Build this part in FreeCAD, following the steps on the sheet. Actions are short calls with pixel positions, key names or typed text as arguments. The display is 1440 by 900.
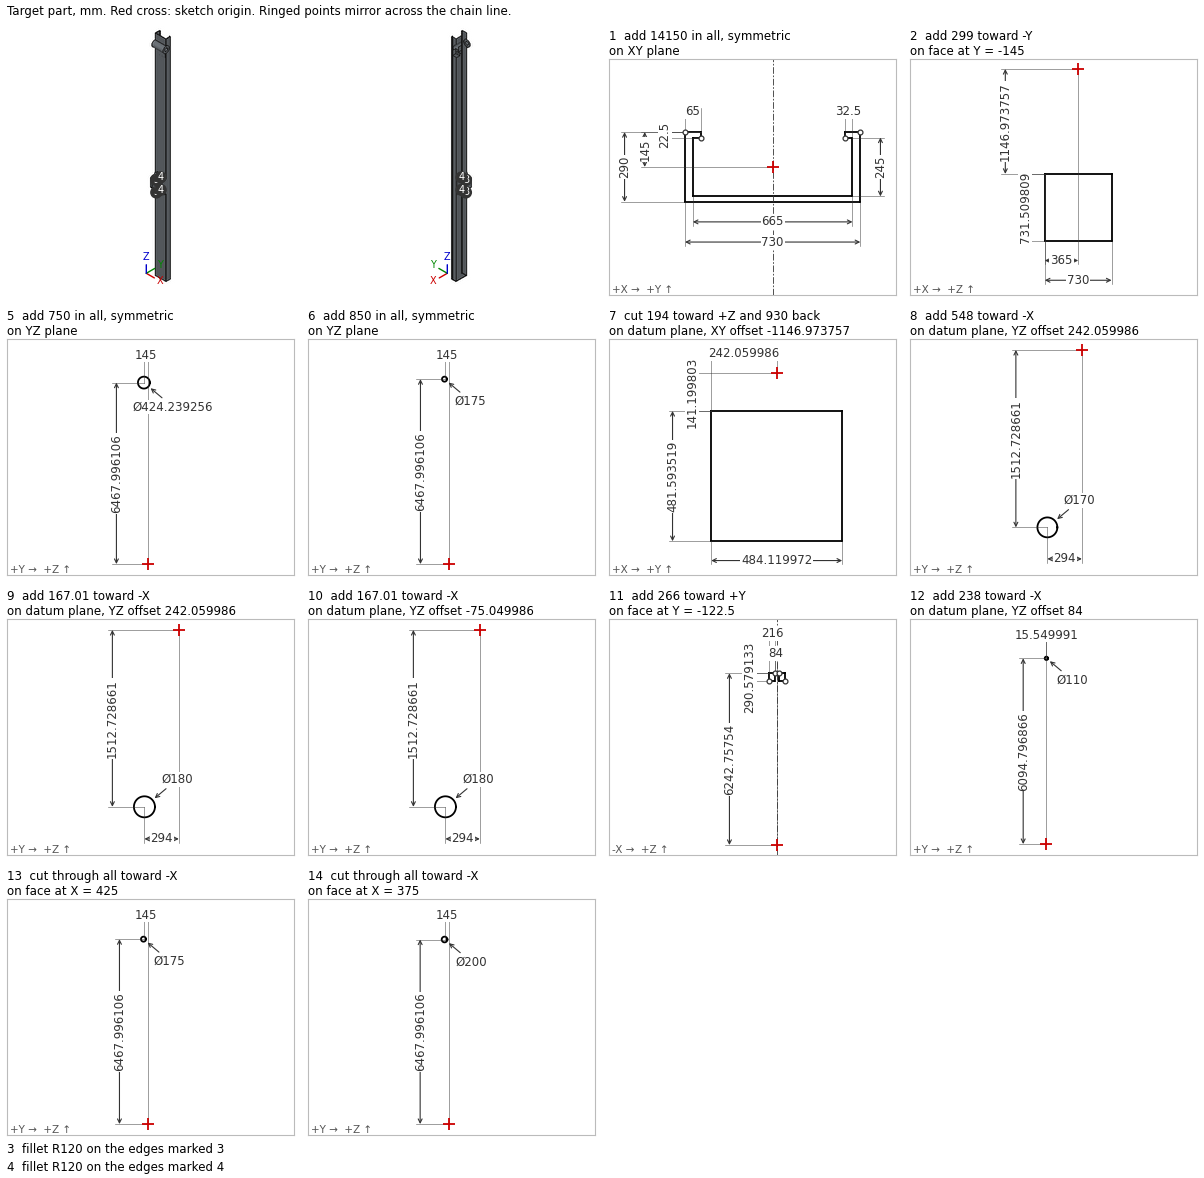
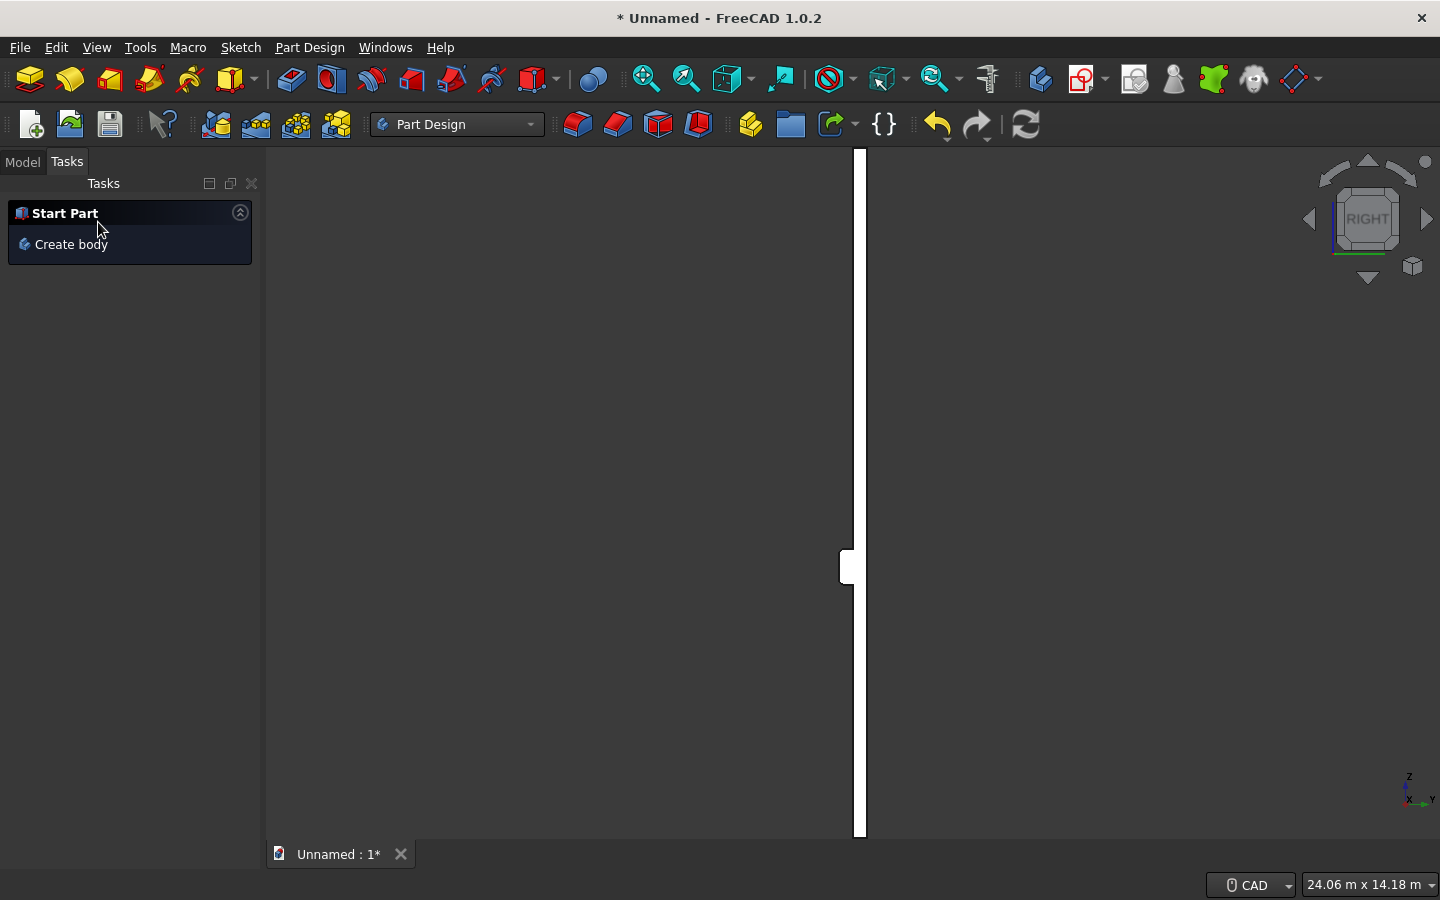
key(5)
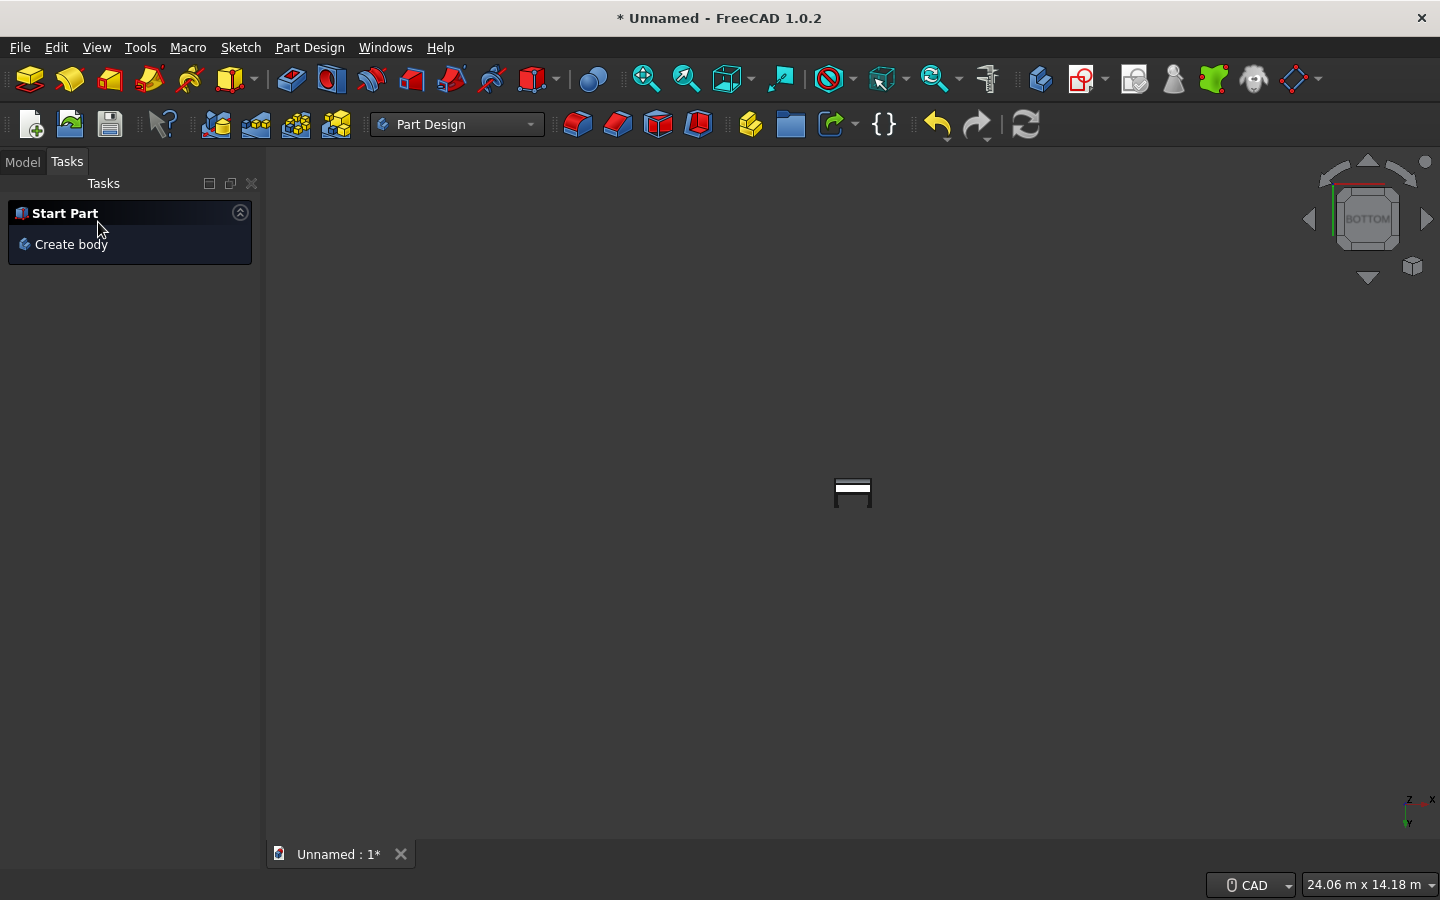
key(v)
key(f)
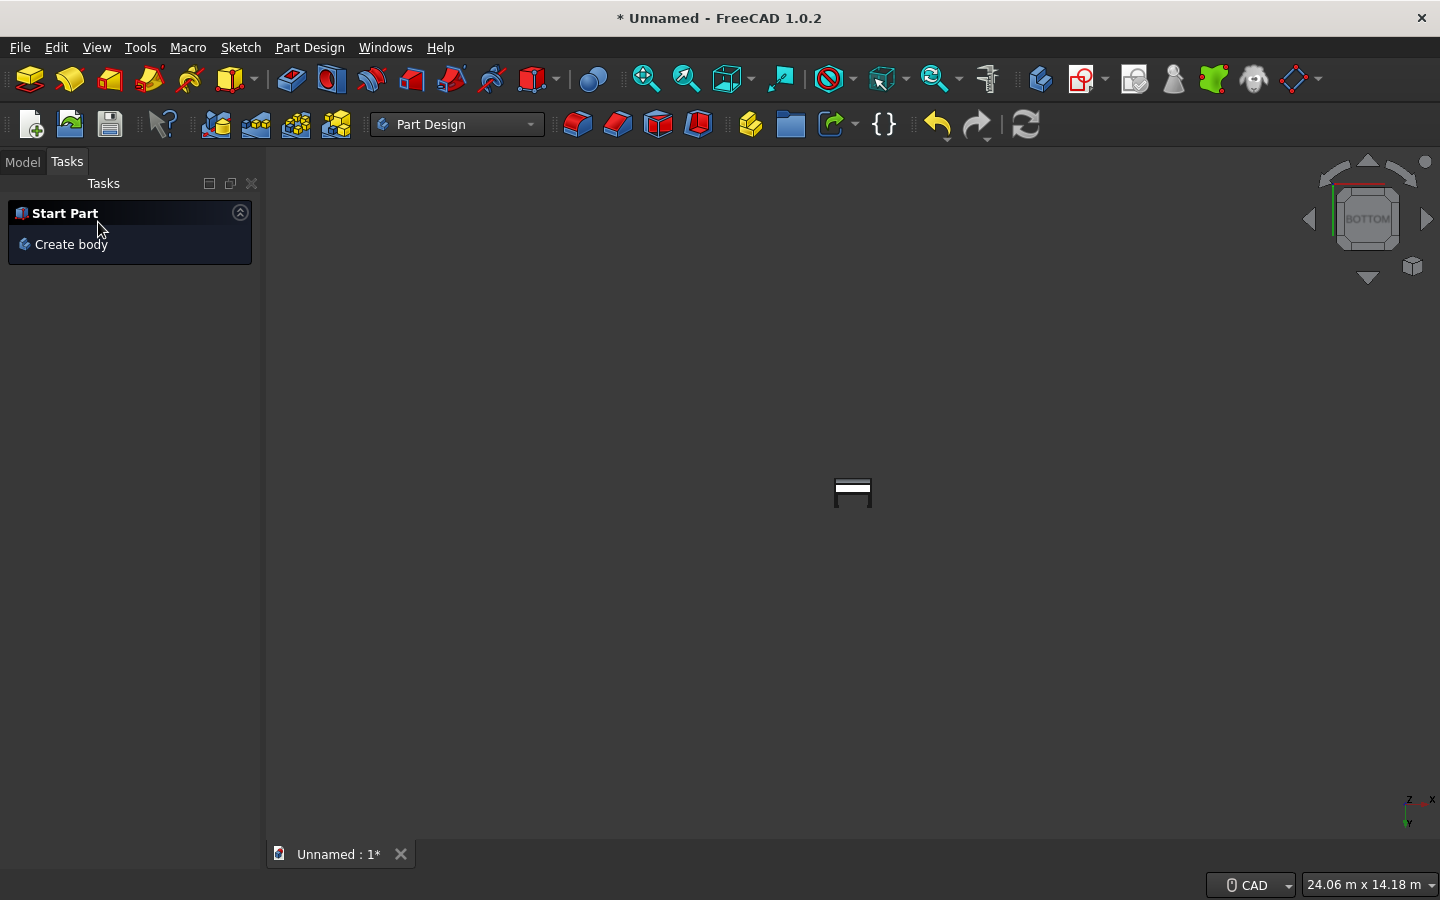
key(4)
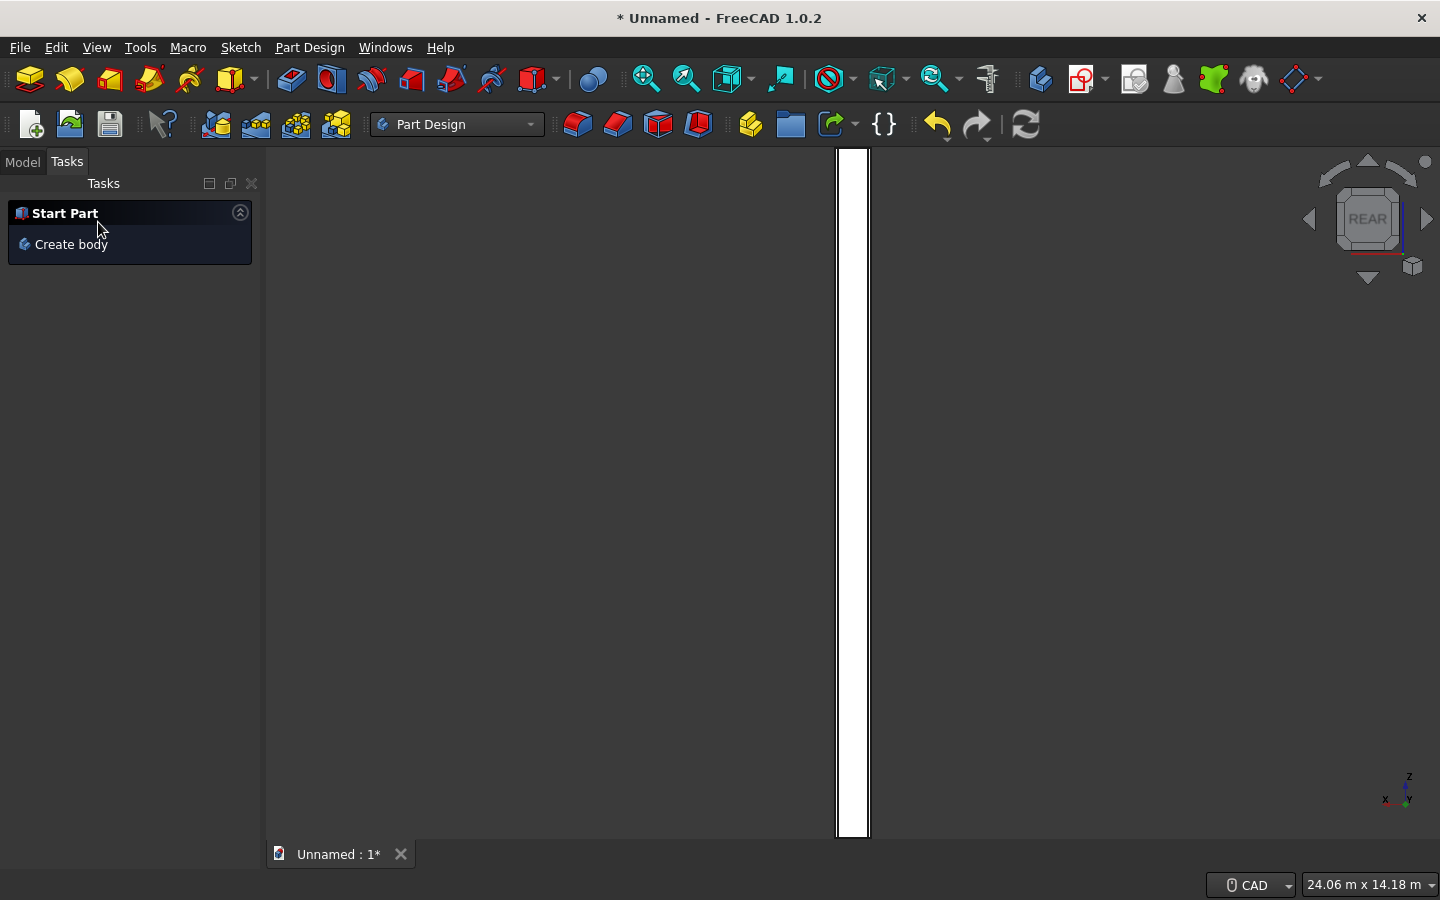
key(6)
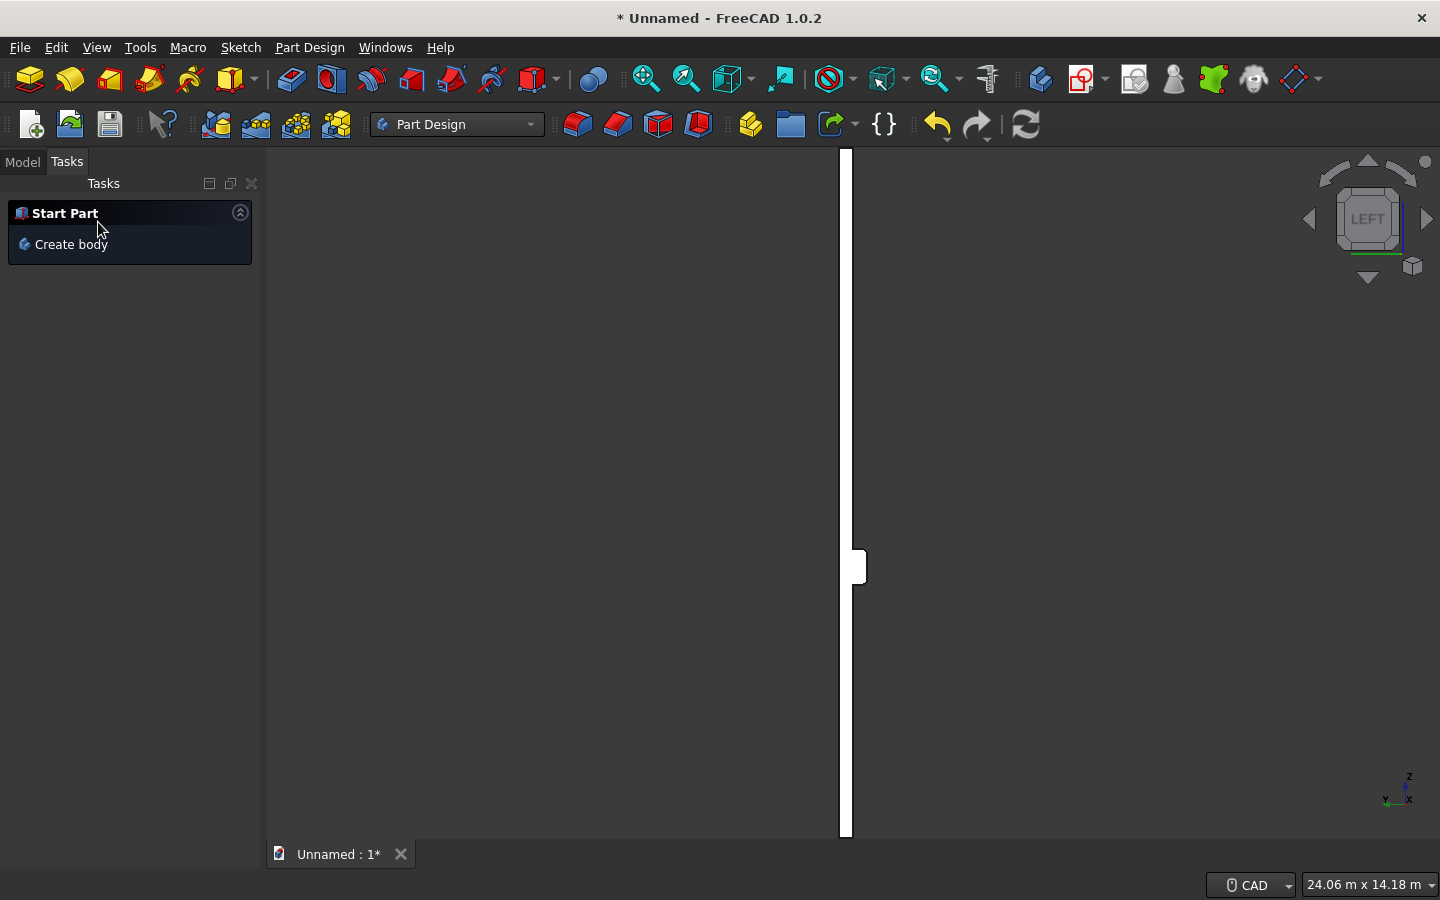
key(v)
key(3)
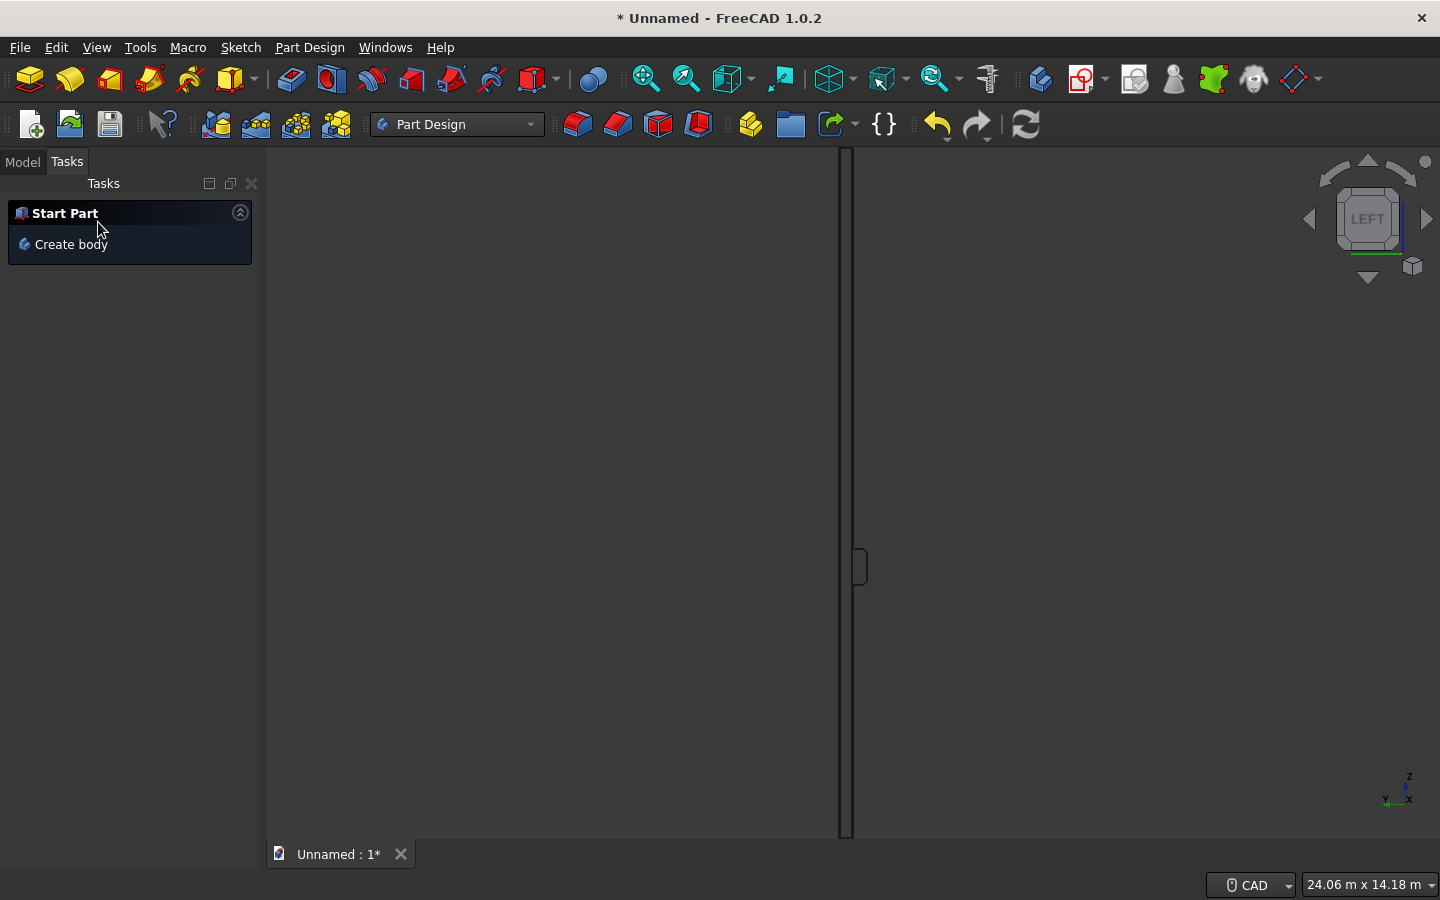
key(0)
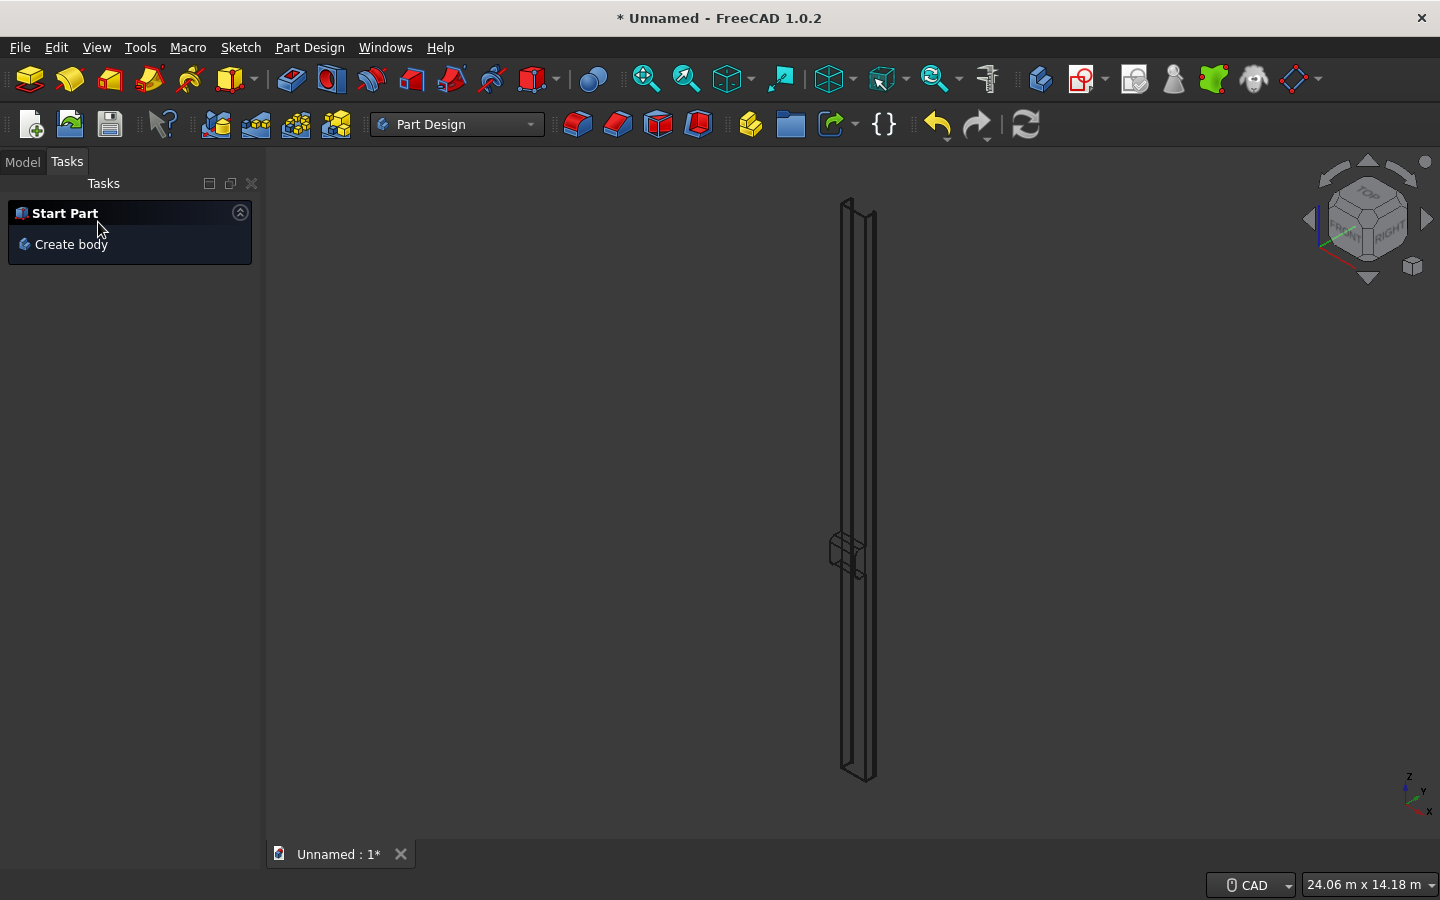
click(856, 539)